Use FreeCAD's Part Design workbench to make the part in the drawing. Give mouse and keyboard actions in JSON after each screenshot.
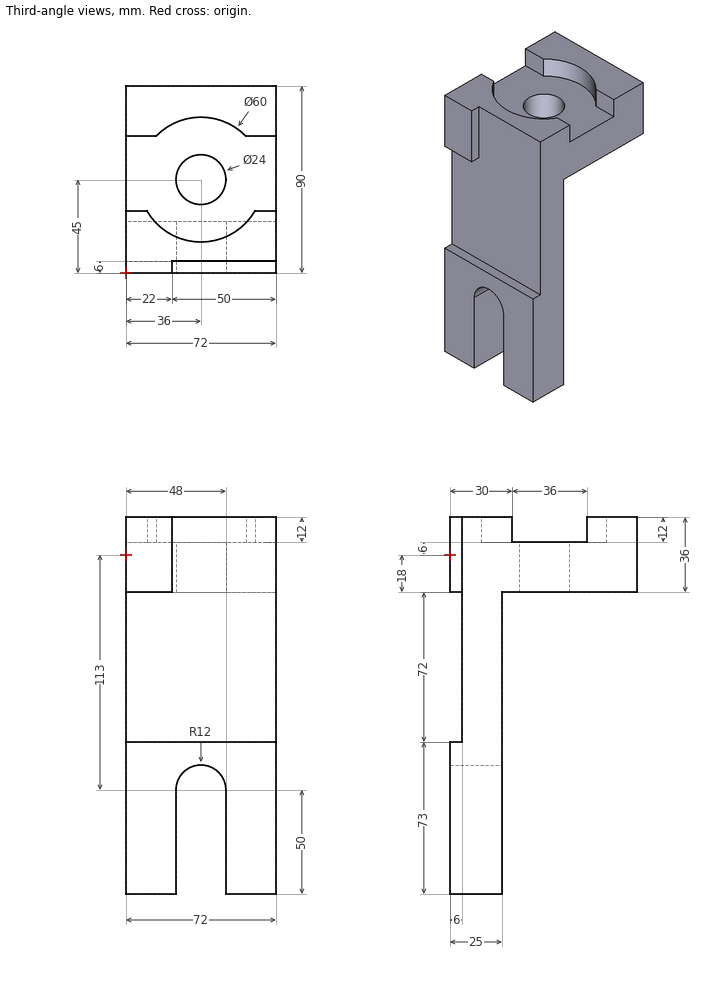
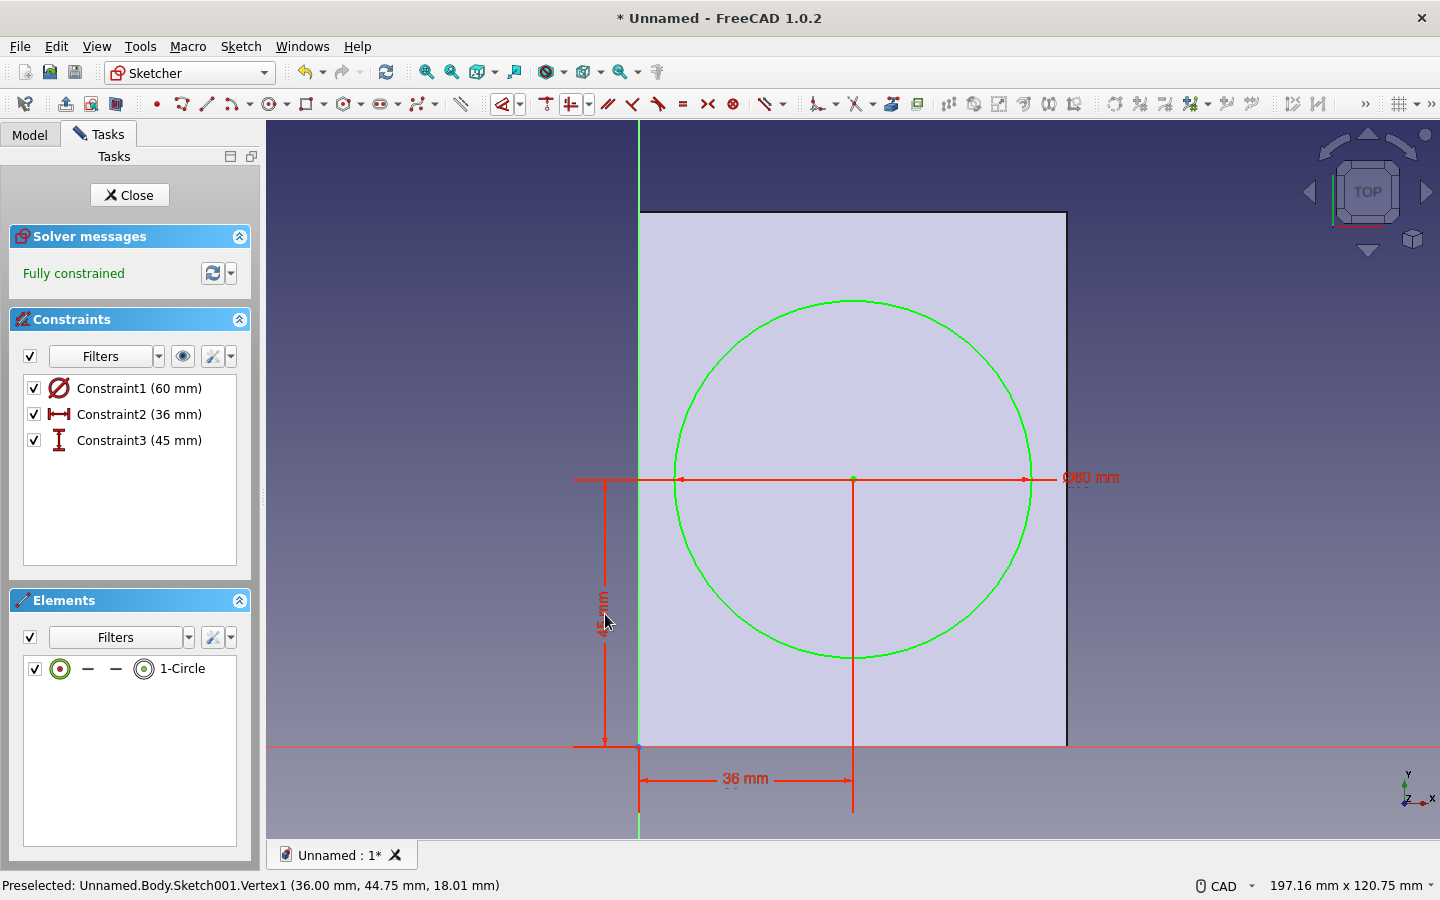
{"action": "left_click", "coordinate": [130, 195]}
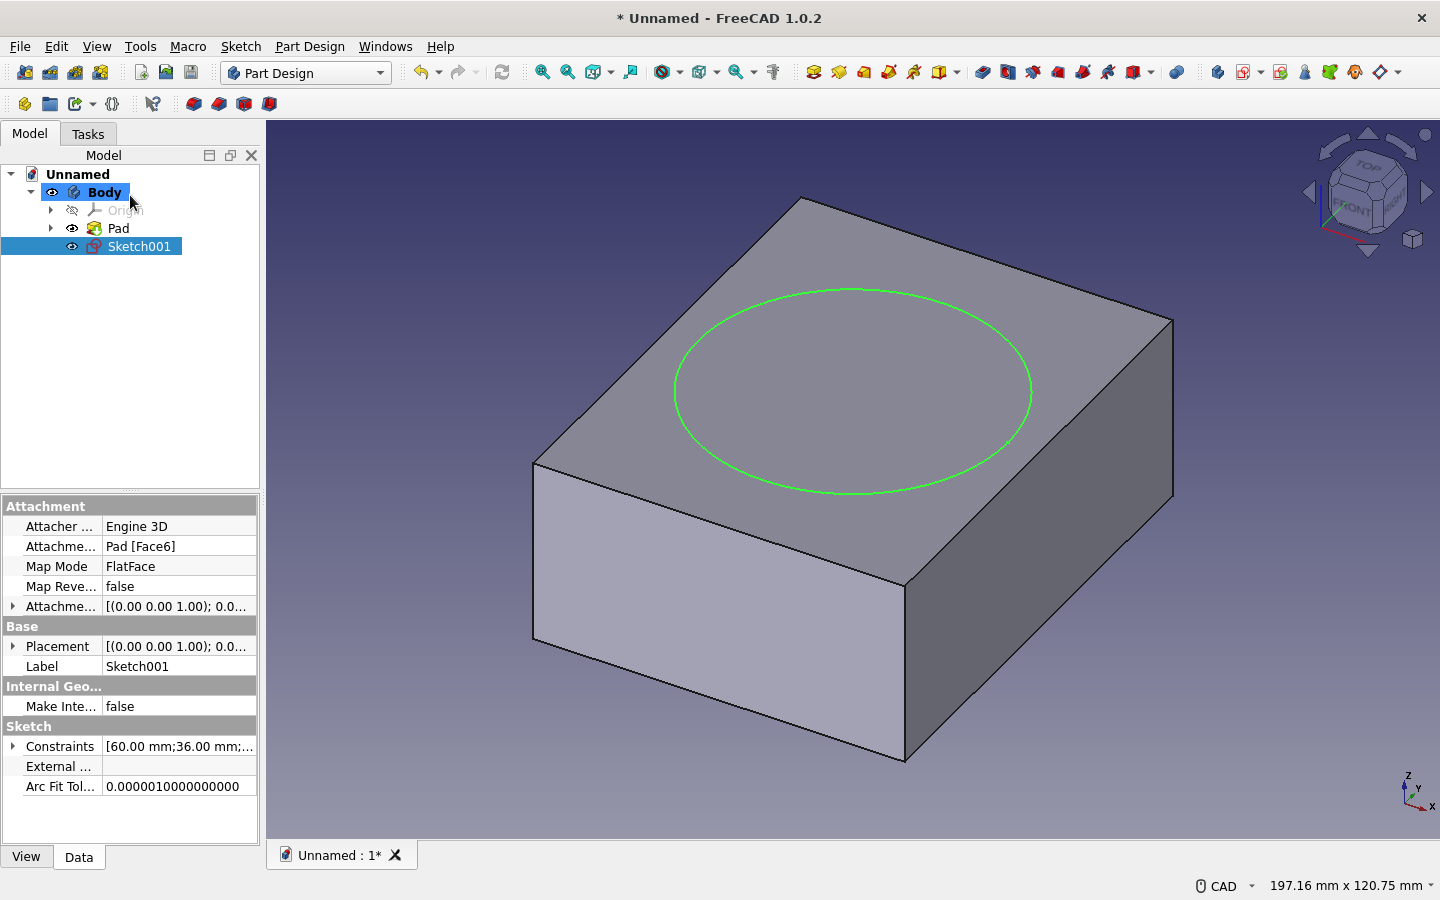
{"action": "left_click", "coordinate": [983, 72]}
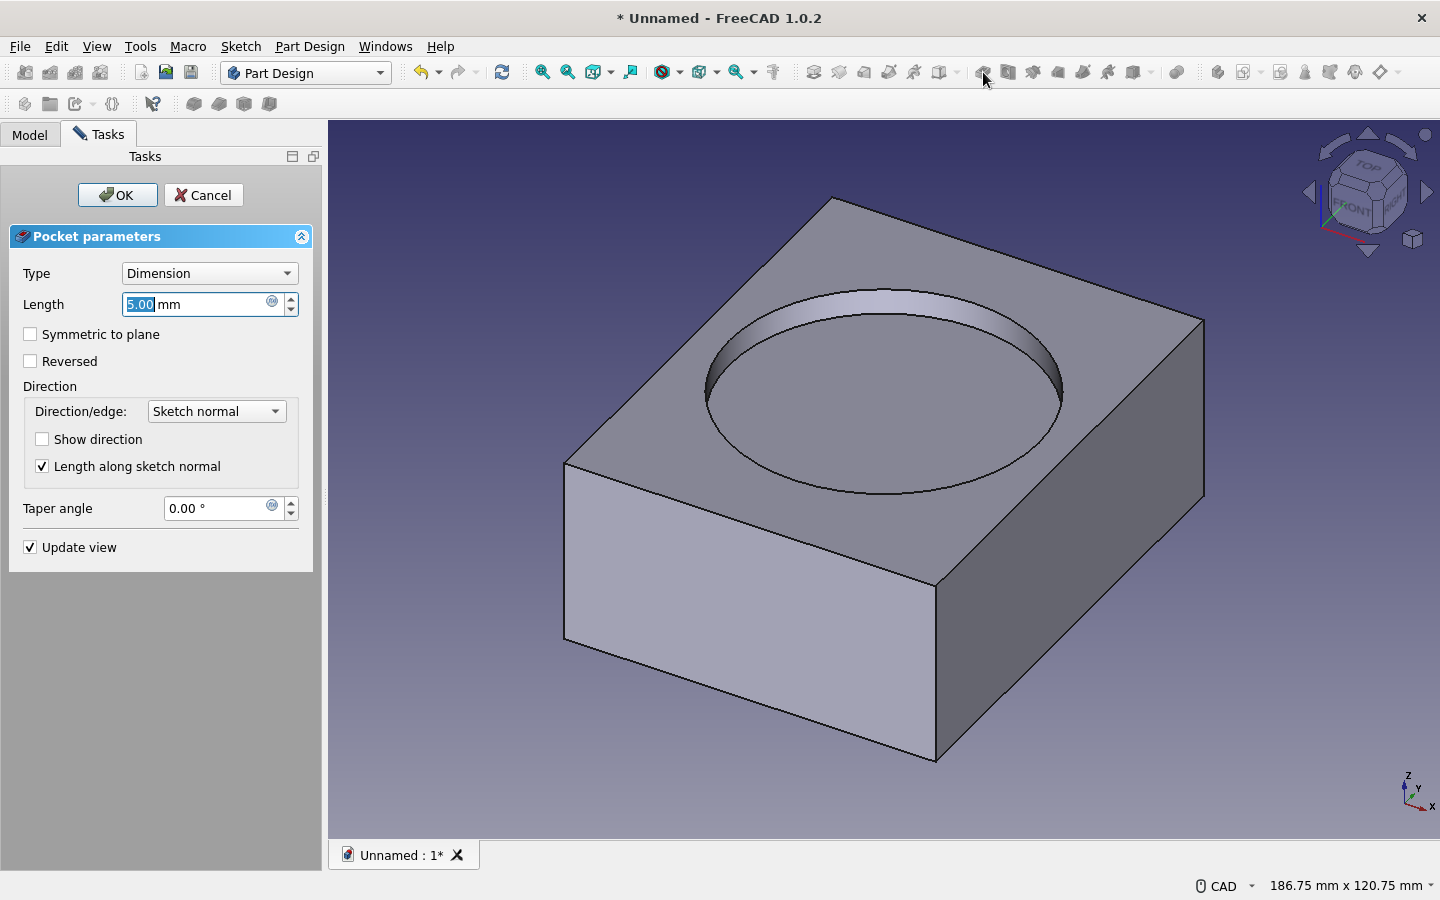
{"action": "type", "text": "12"}
{"action": "key", "text": "Tab"}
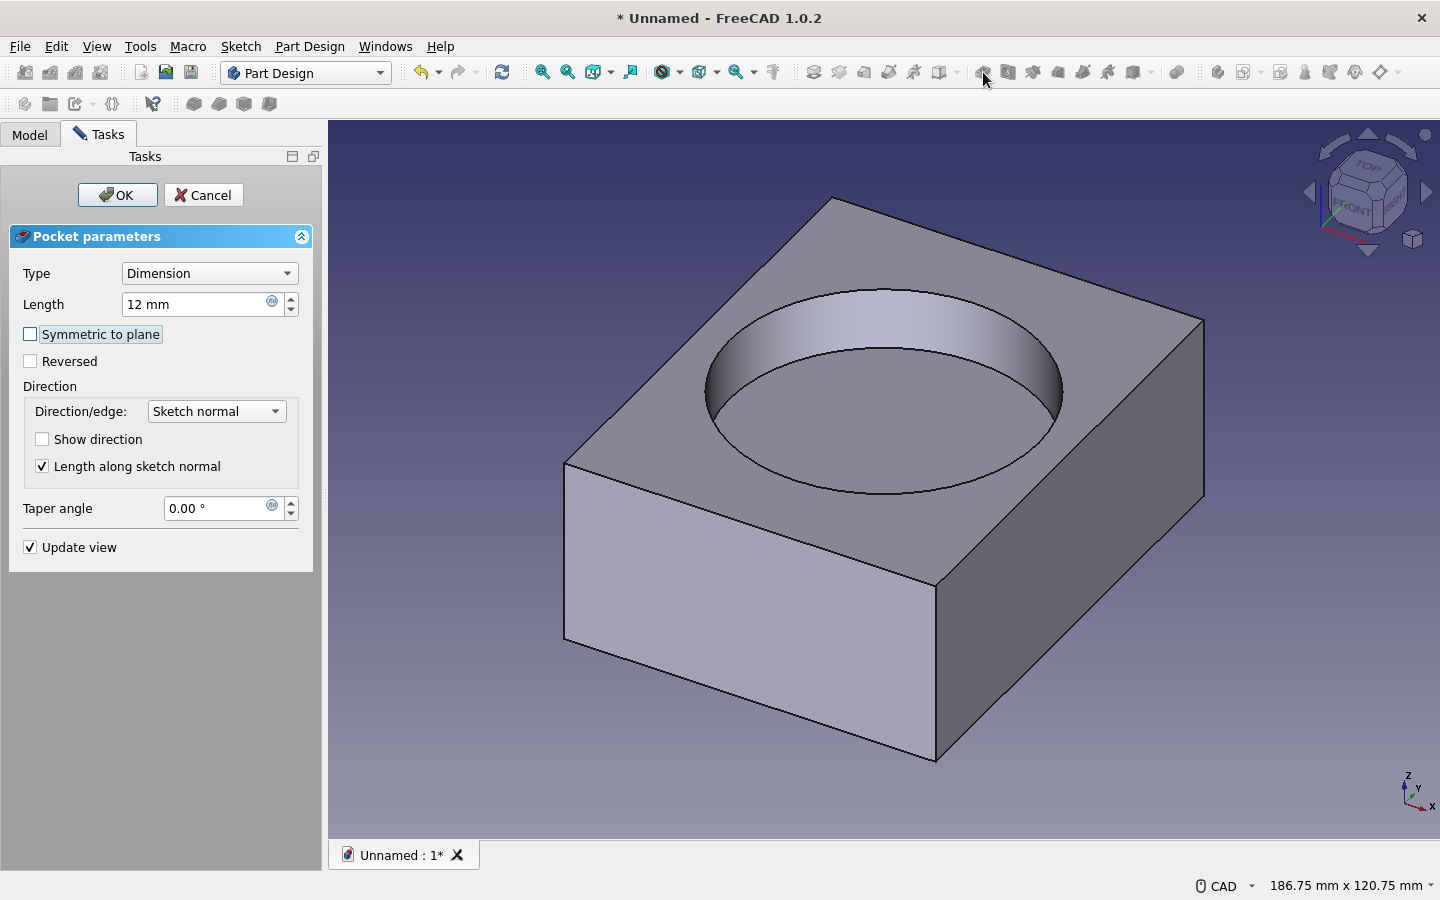
{"action": "left_click", "coordinate": [118, 195]}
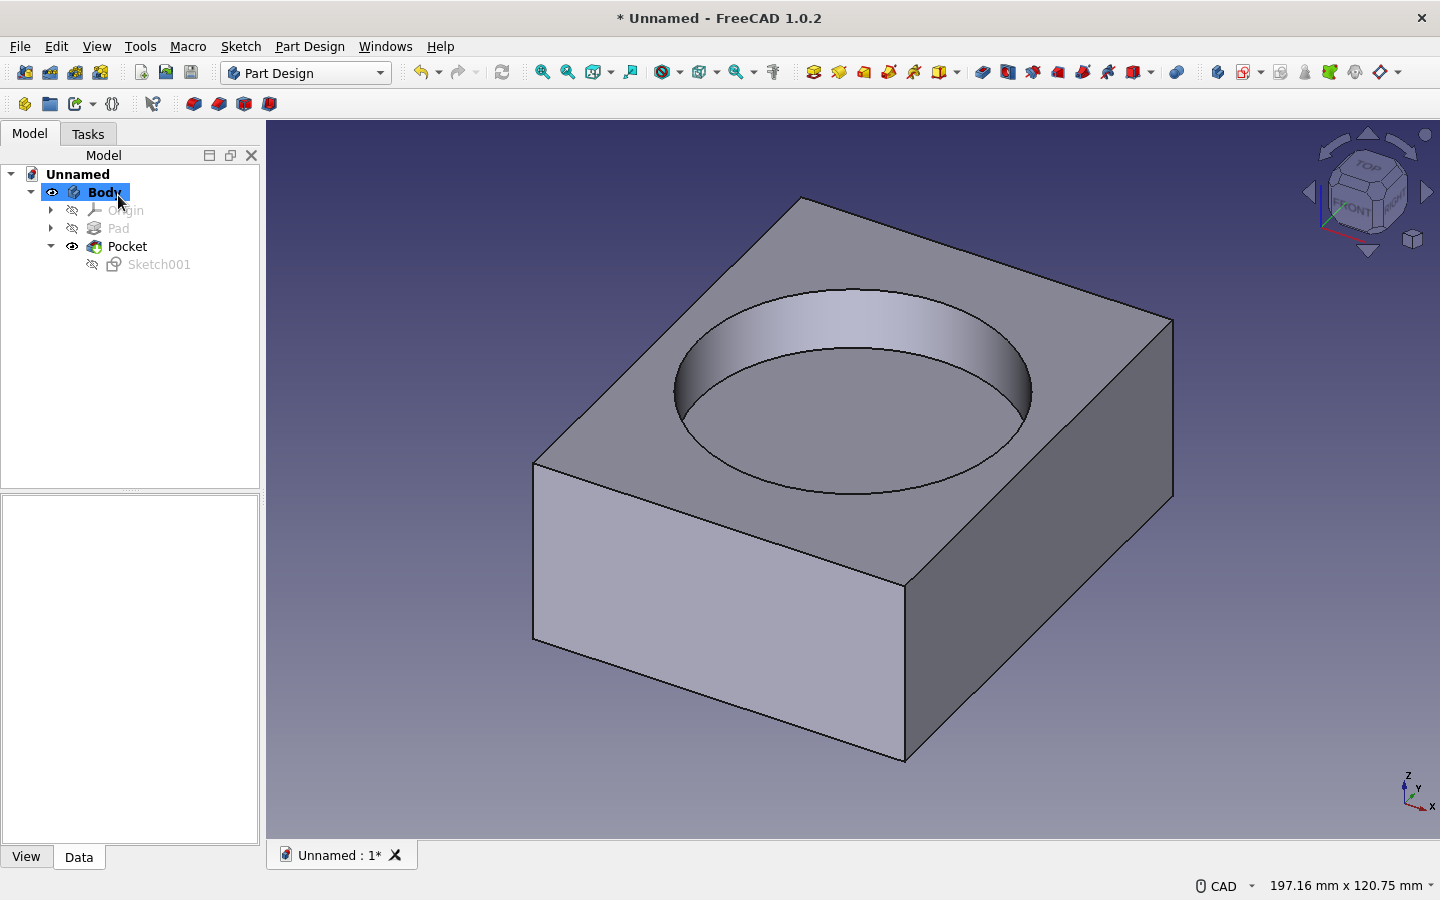
{"action": "left_click", "coordinate": [1115, 464]}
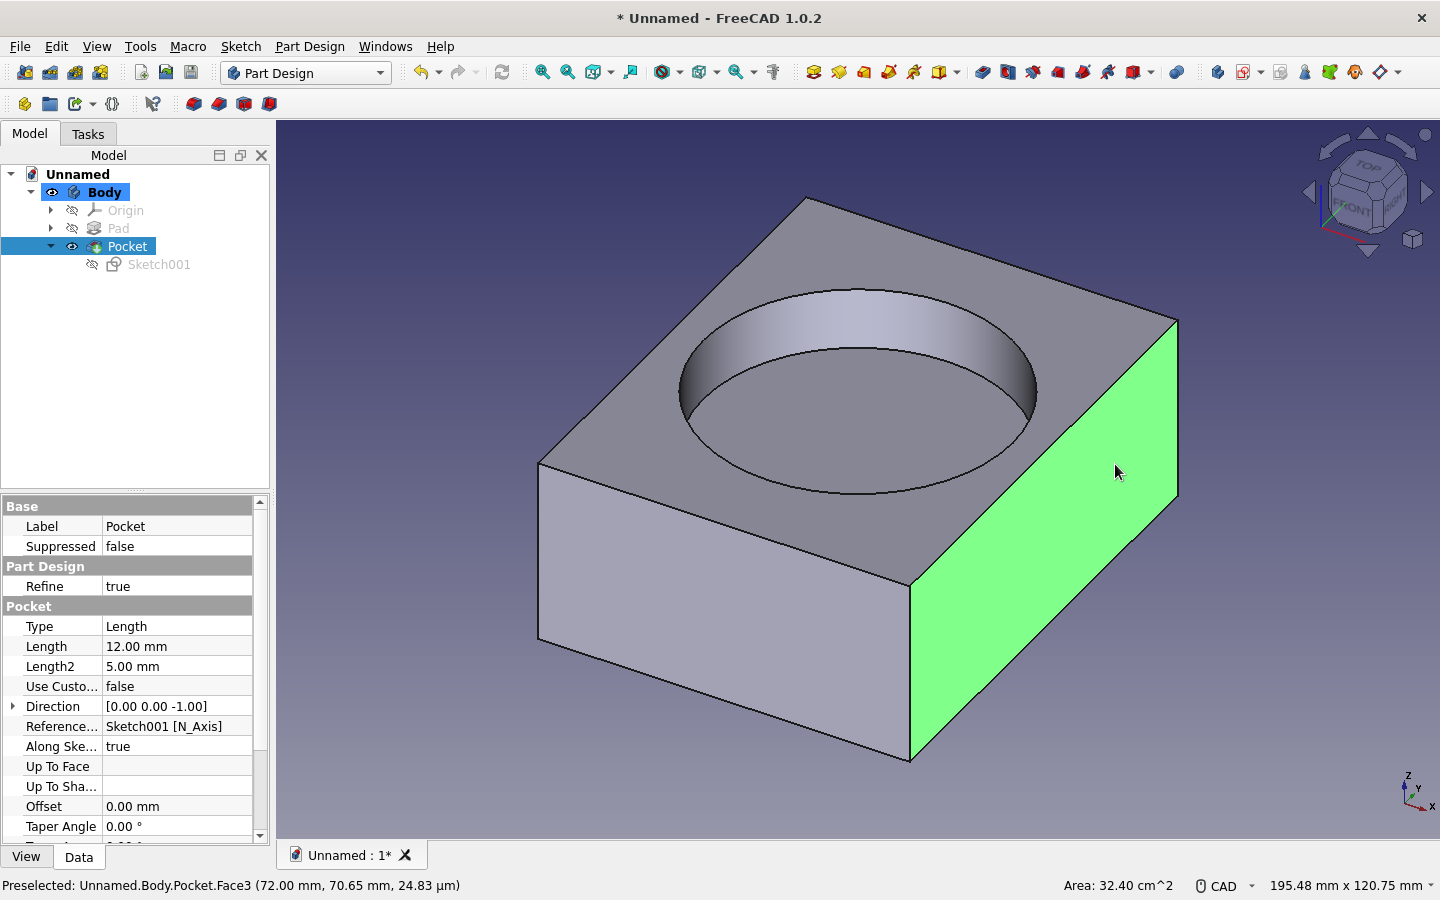
{"action": "left_click", "coordinate": [1242, 72]}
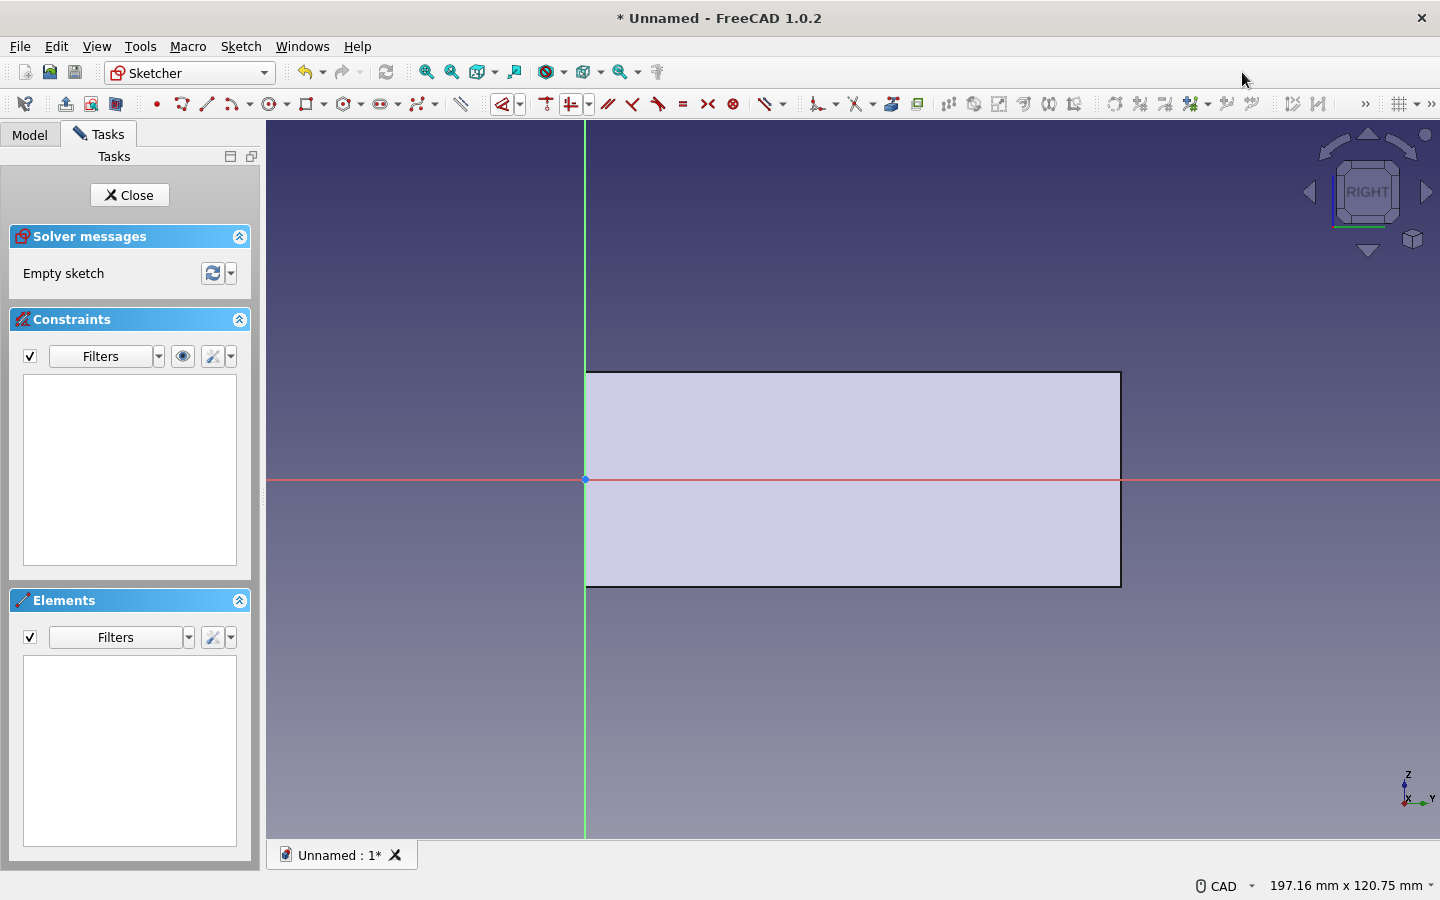
{"action": "scroll", "coordinate": [778, 361], "scroll_direction": "up", "scroll_amount": 3}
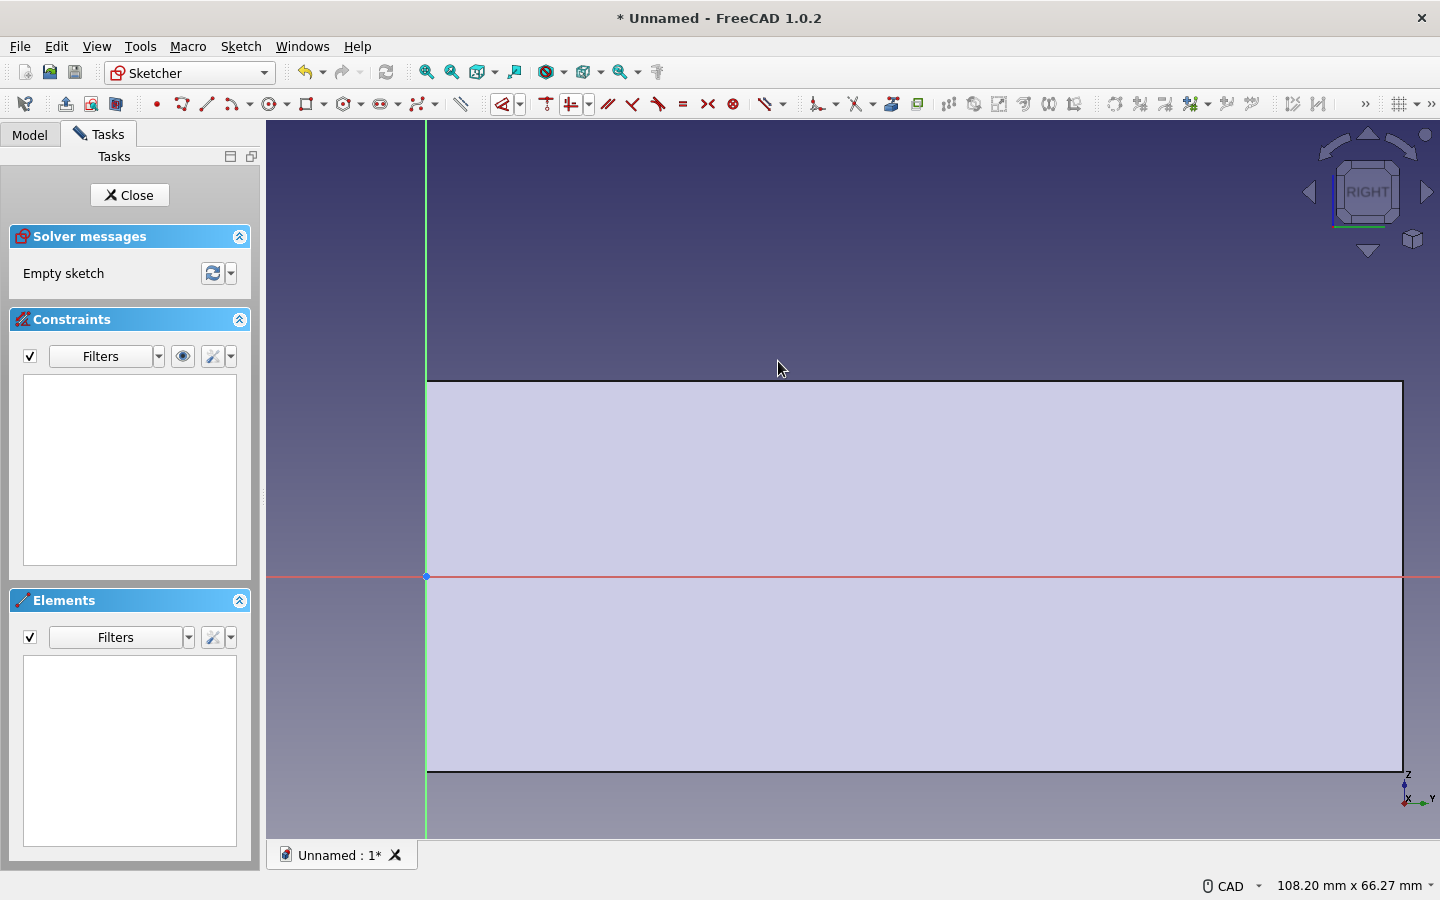
{"action": "key", "text": "g r"}